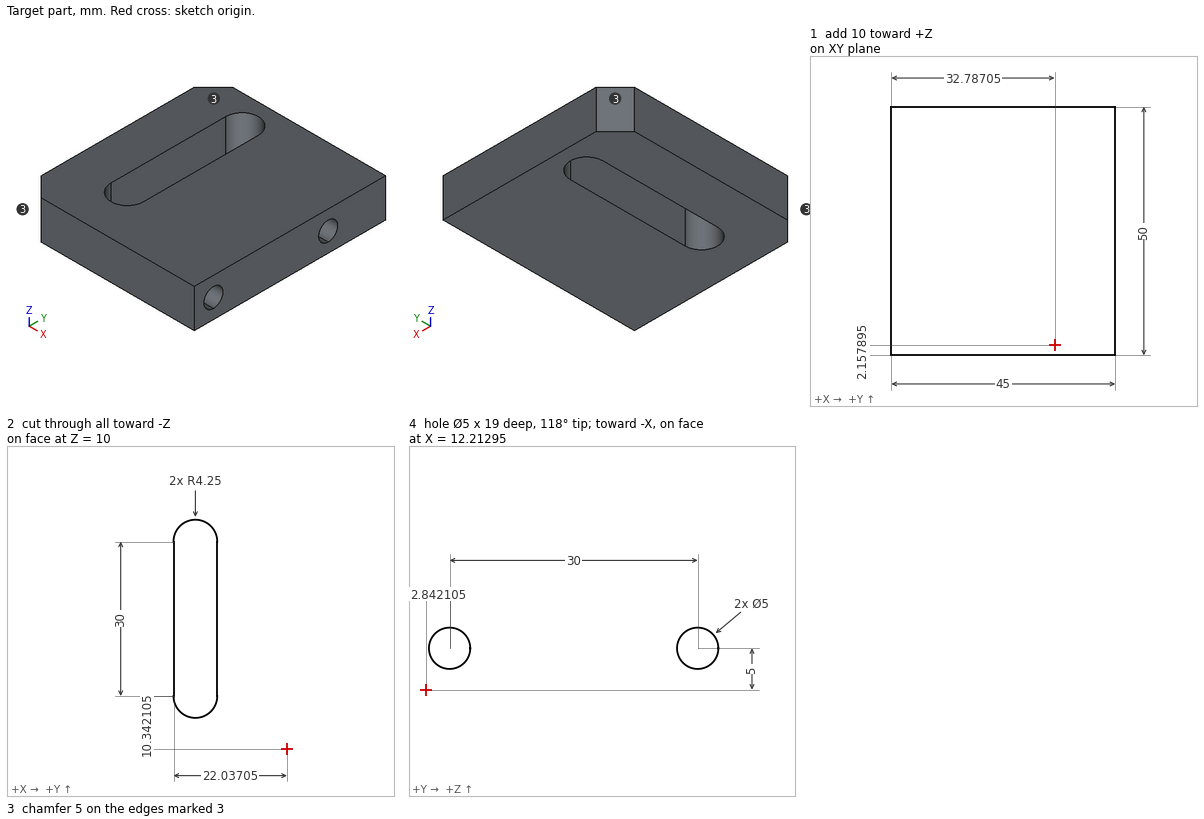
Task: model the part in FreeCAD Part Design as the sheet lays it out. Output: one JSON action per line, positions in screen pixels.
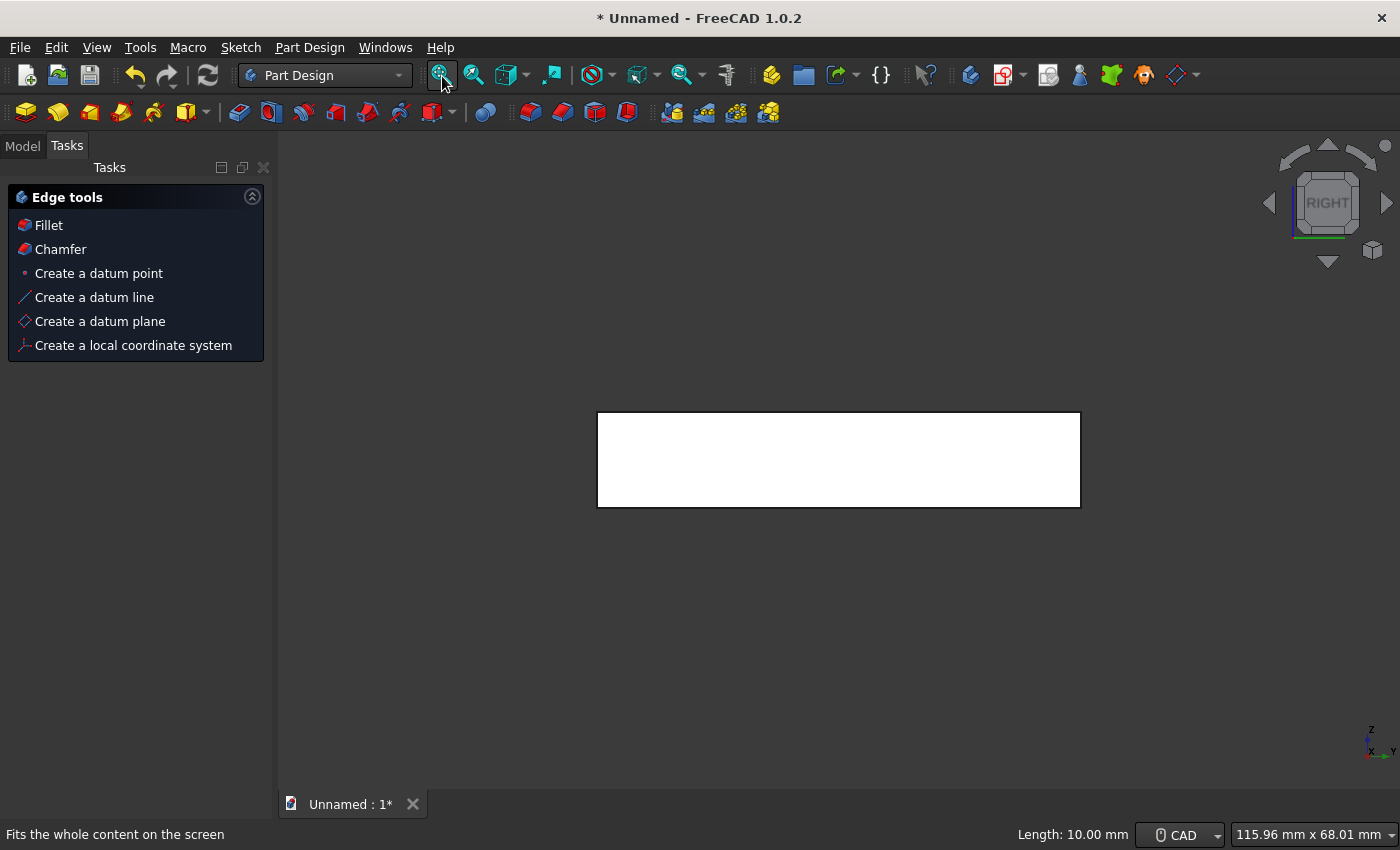
{"action": "key", "text": "5"}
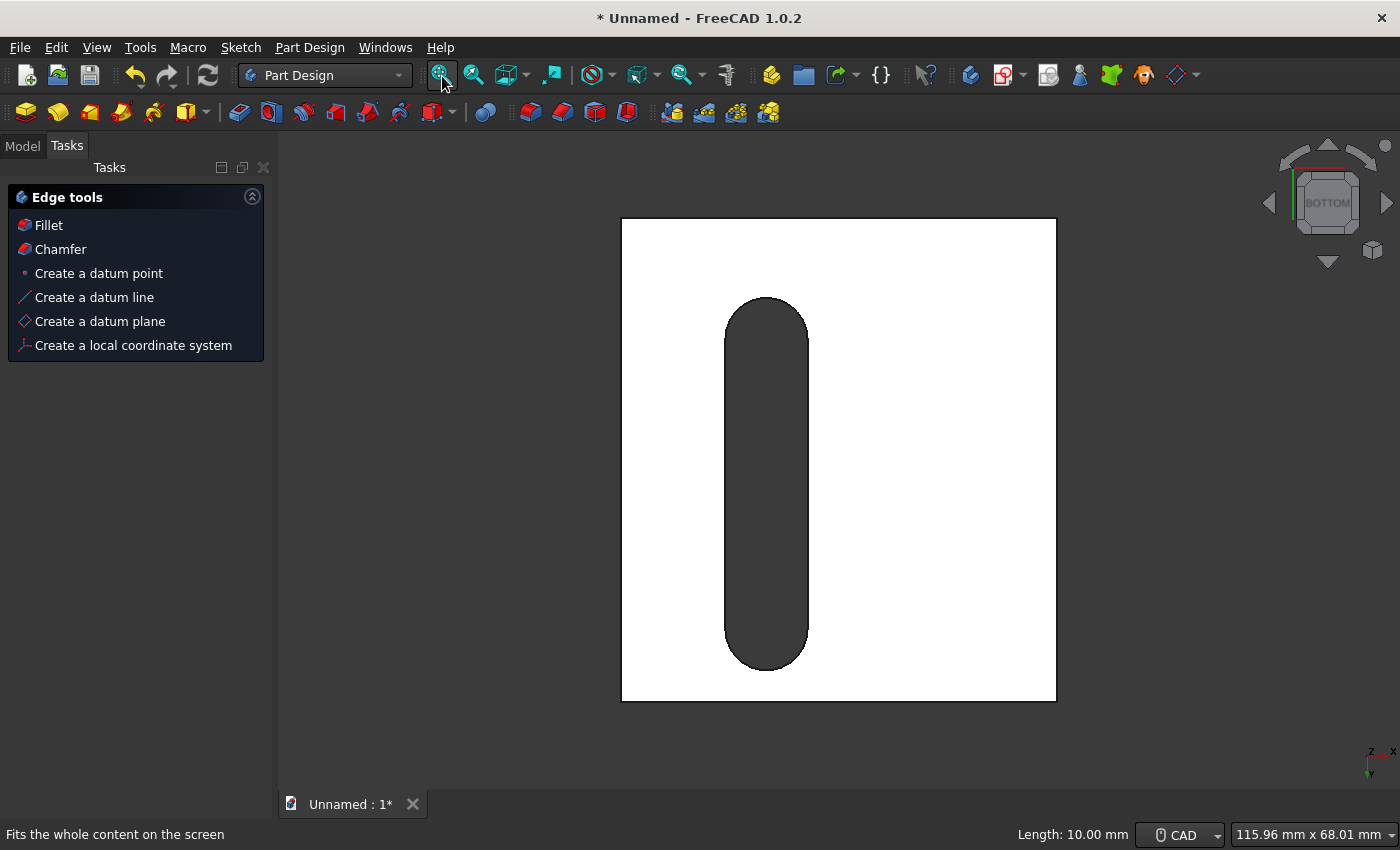
{"action": "key", "text": "4"}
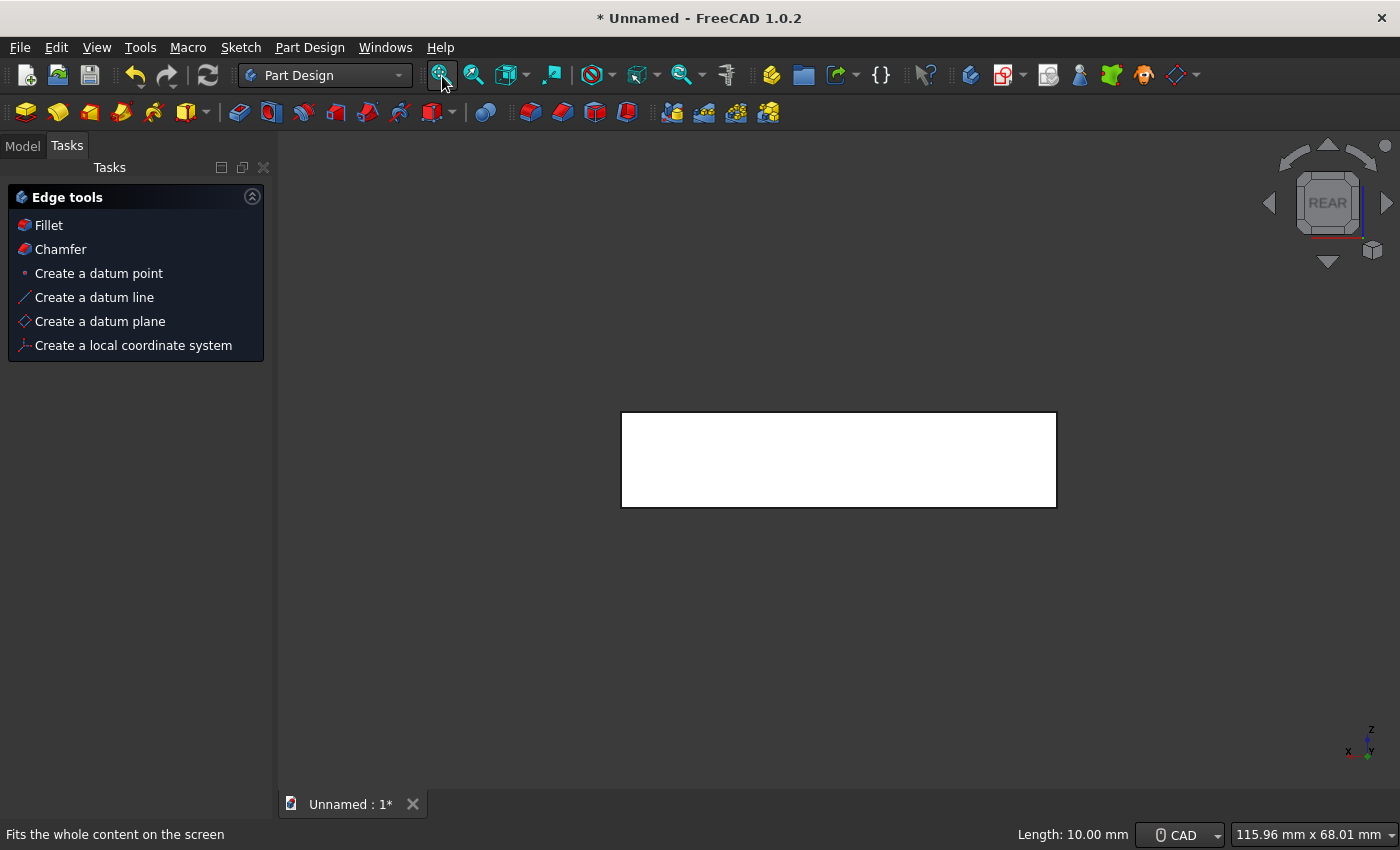
{"action": "key", "text": "v f"}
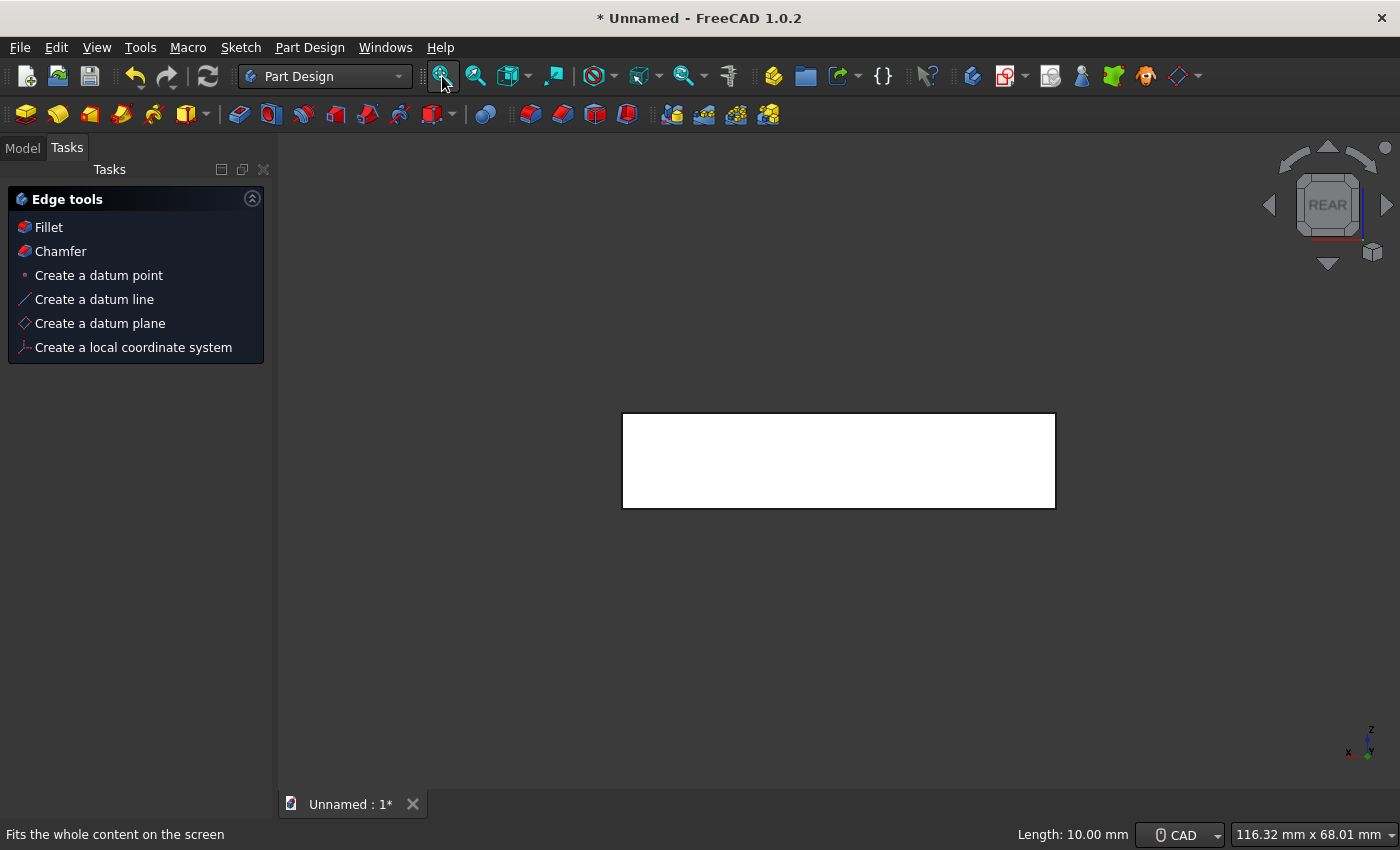
{"action": "left_click", "coordinate": [1056, 460], "text": "ctrl"}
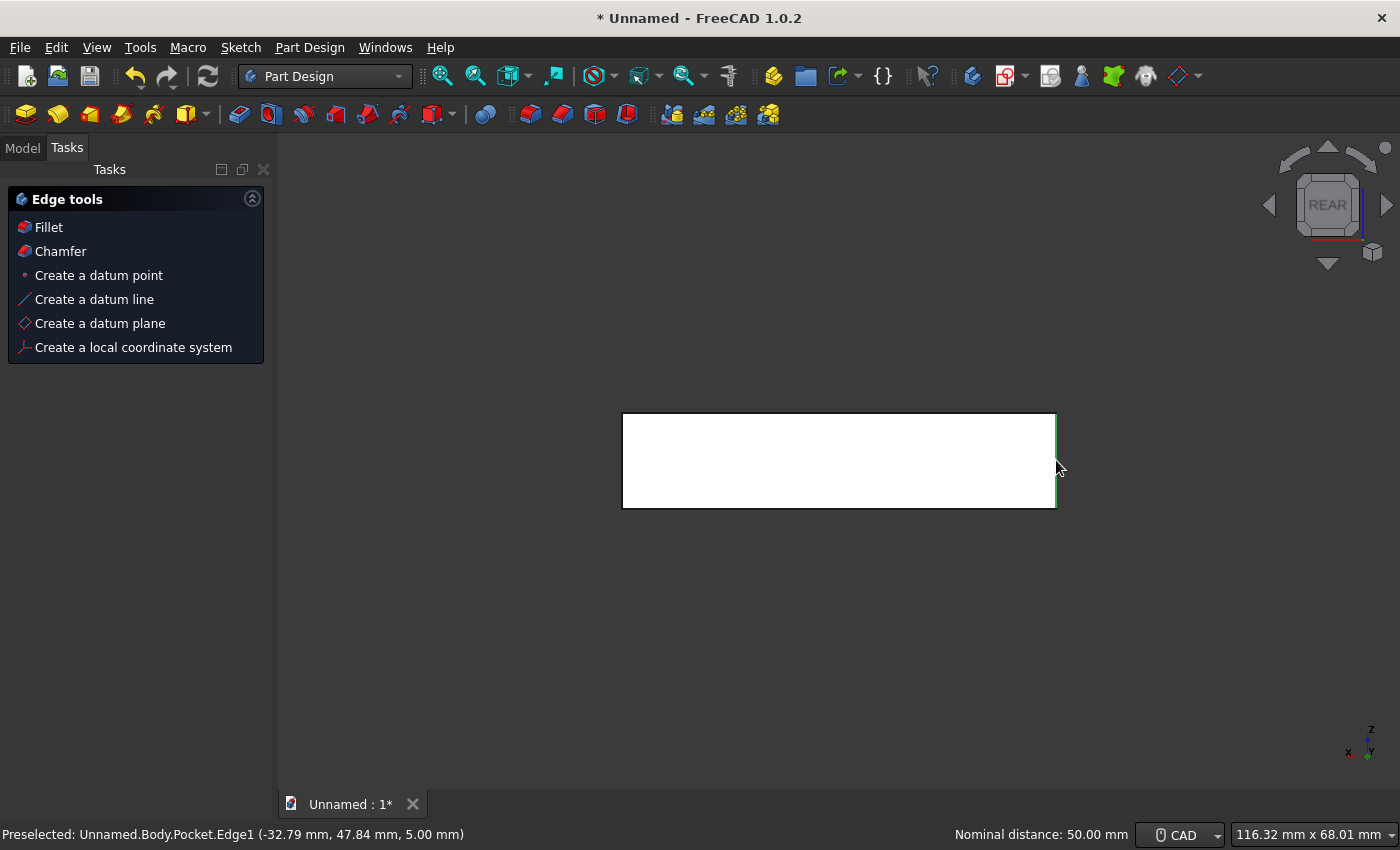
{"action": "left_click", "coordinate": [564, 114]}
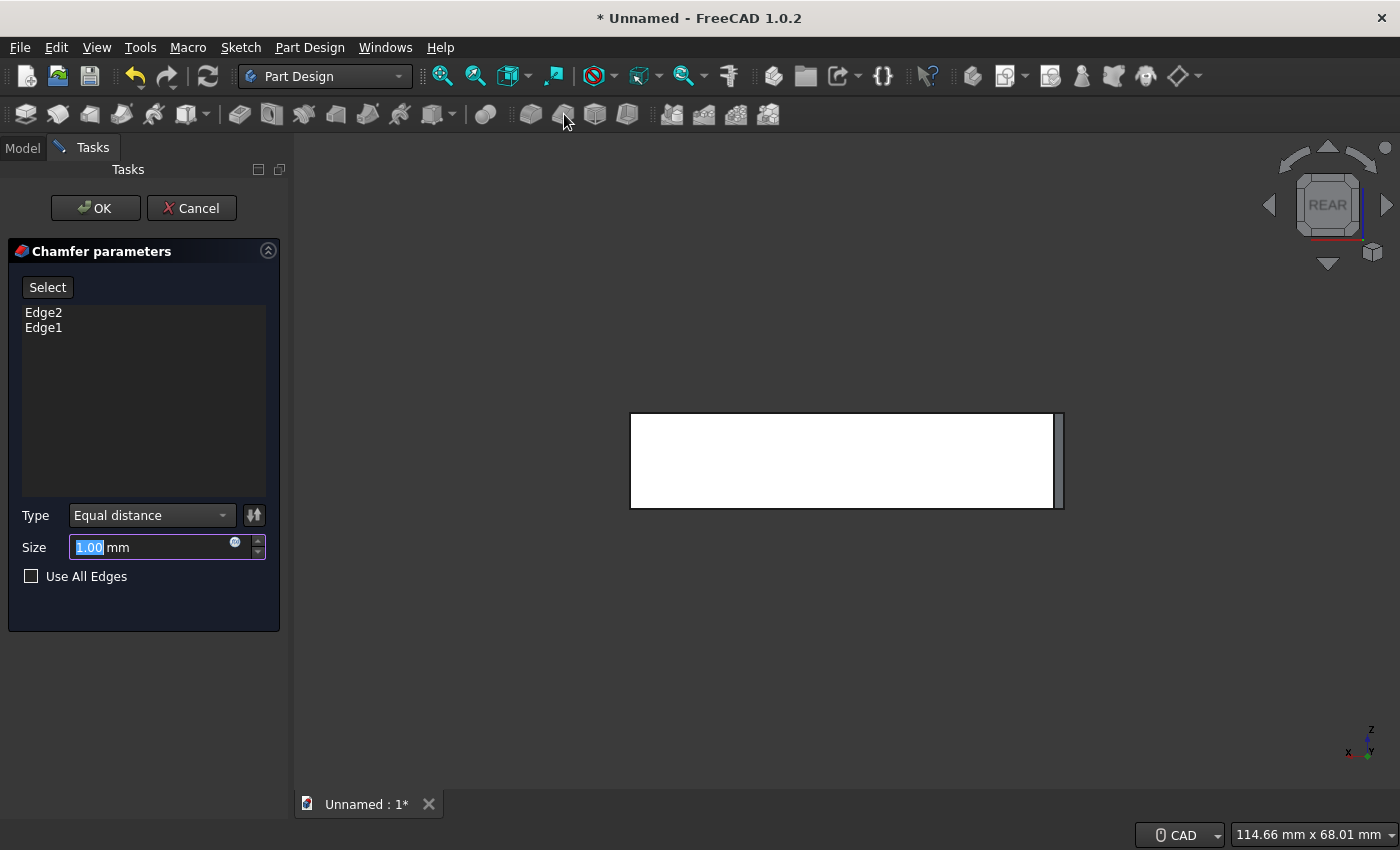
{"action": "type", "text": "5"}
{"action": "key", "text": "Tab"}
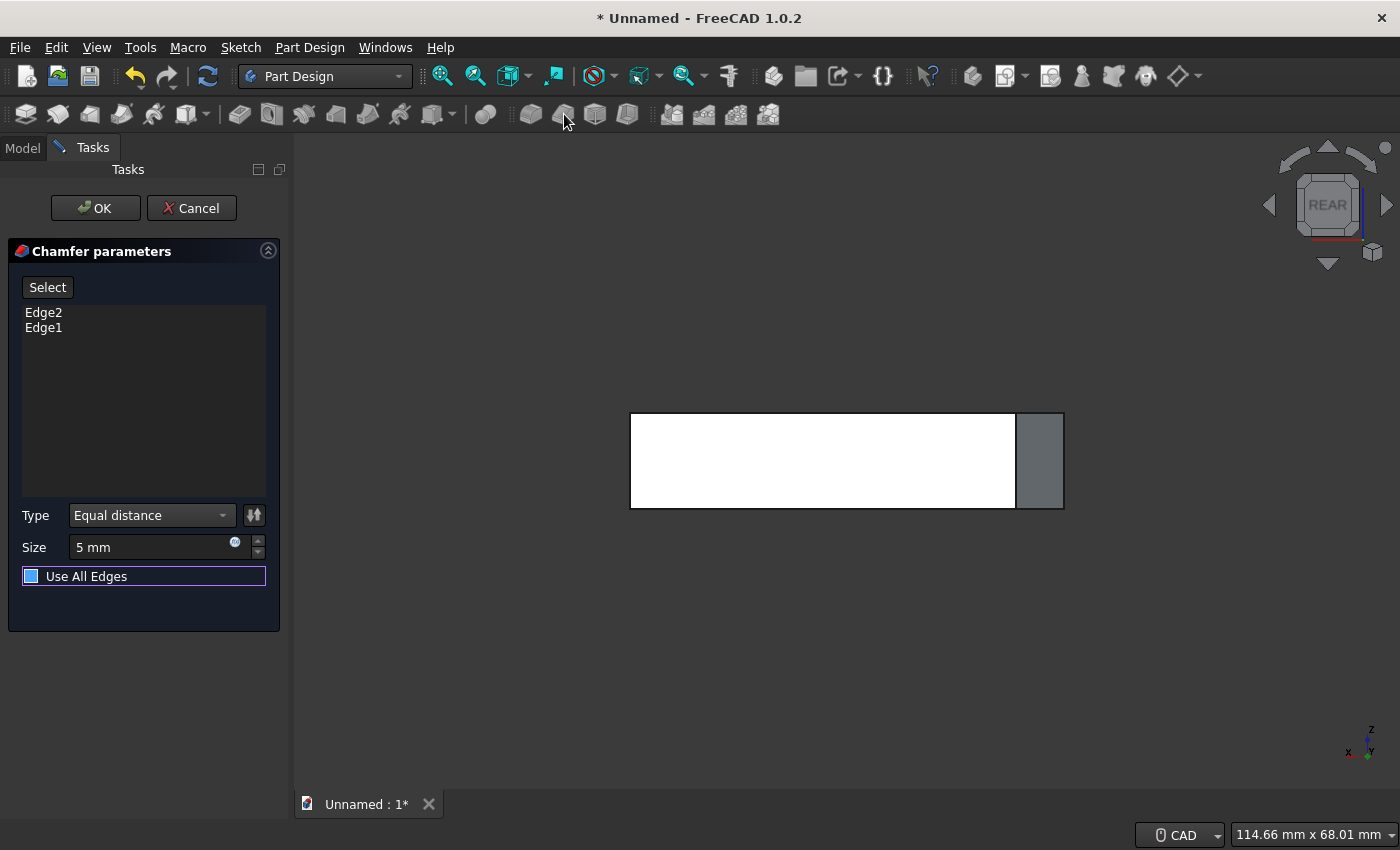
{"action": "left_click", "coordinate": [96, 208]}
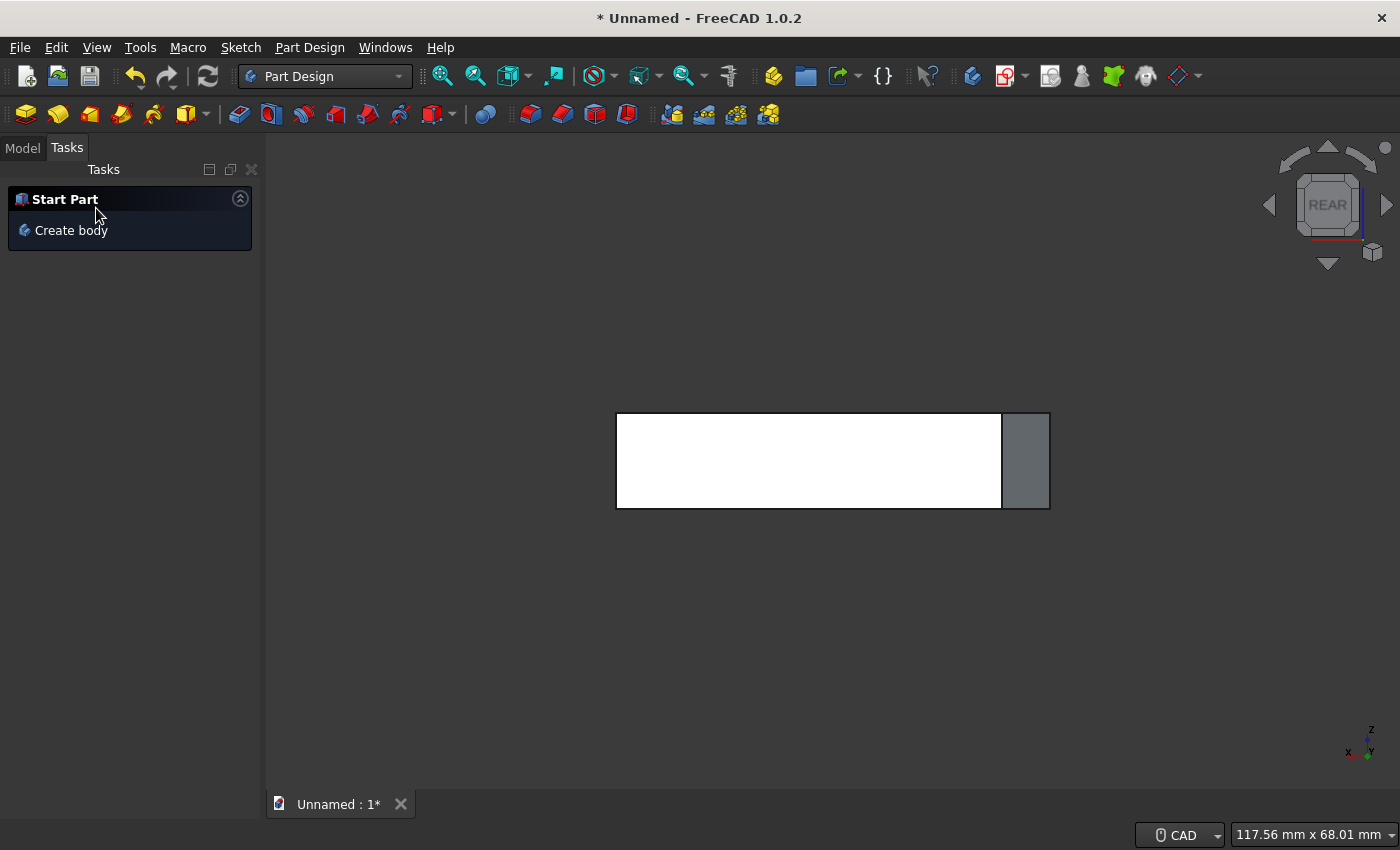
{"action": "key", "text": "v f"}